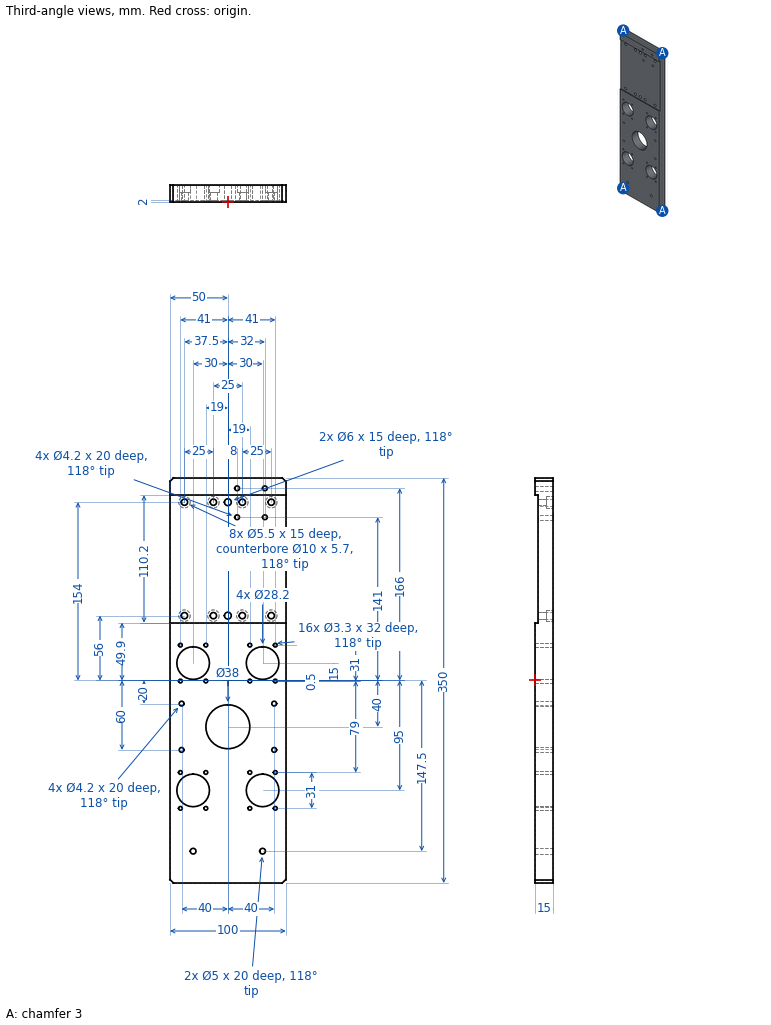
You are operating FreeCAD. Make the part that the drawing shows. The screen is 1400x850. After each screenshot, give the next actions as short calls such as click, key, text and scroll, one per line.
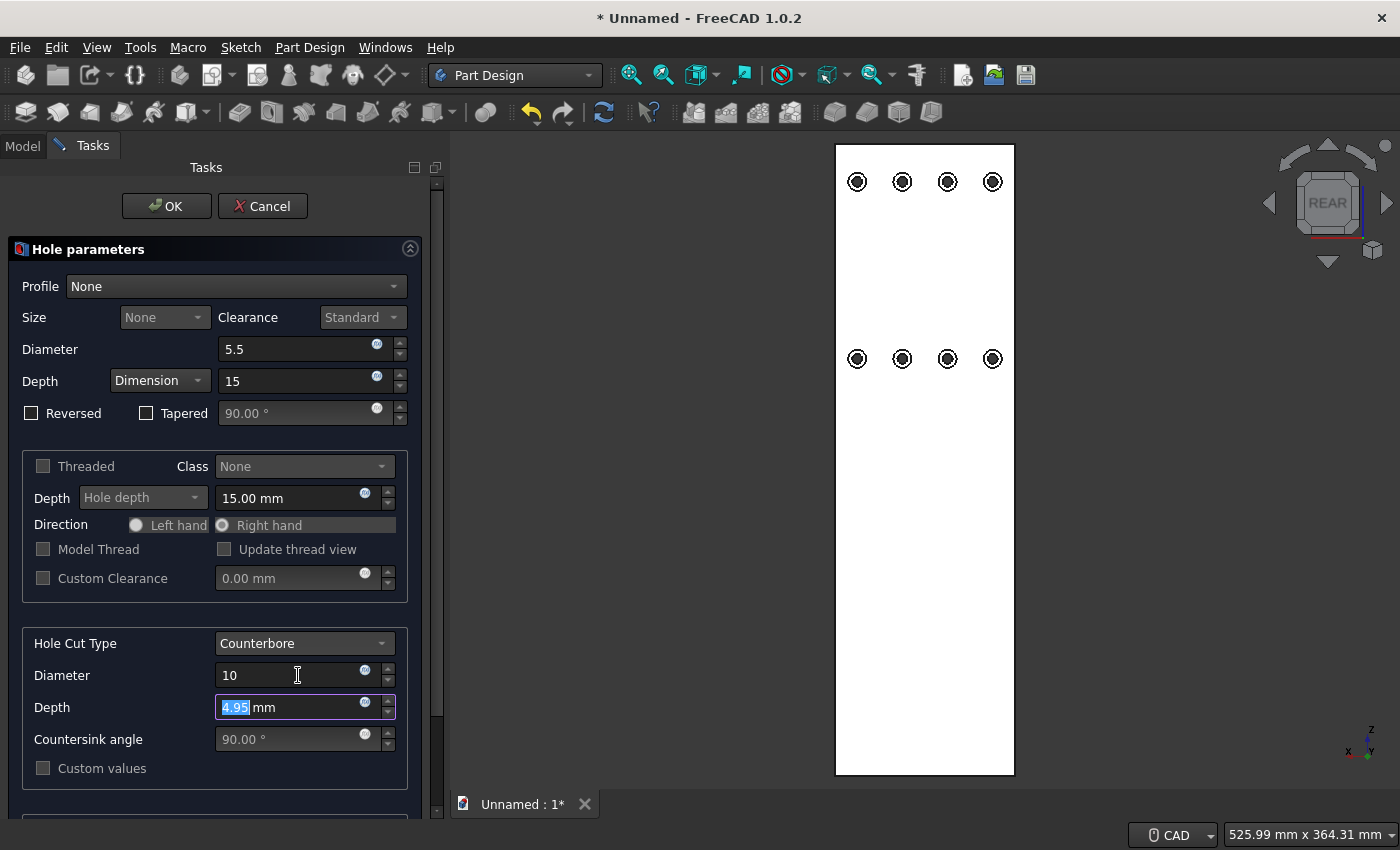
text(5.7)
key(Tab)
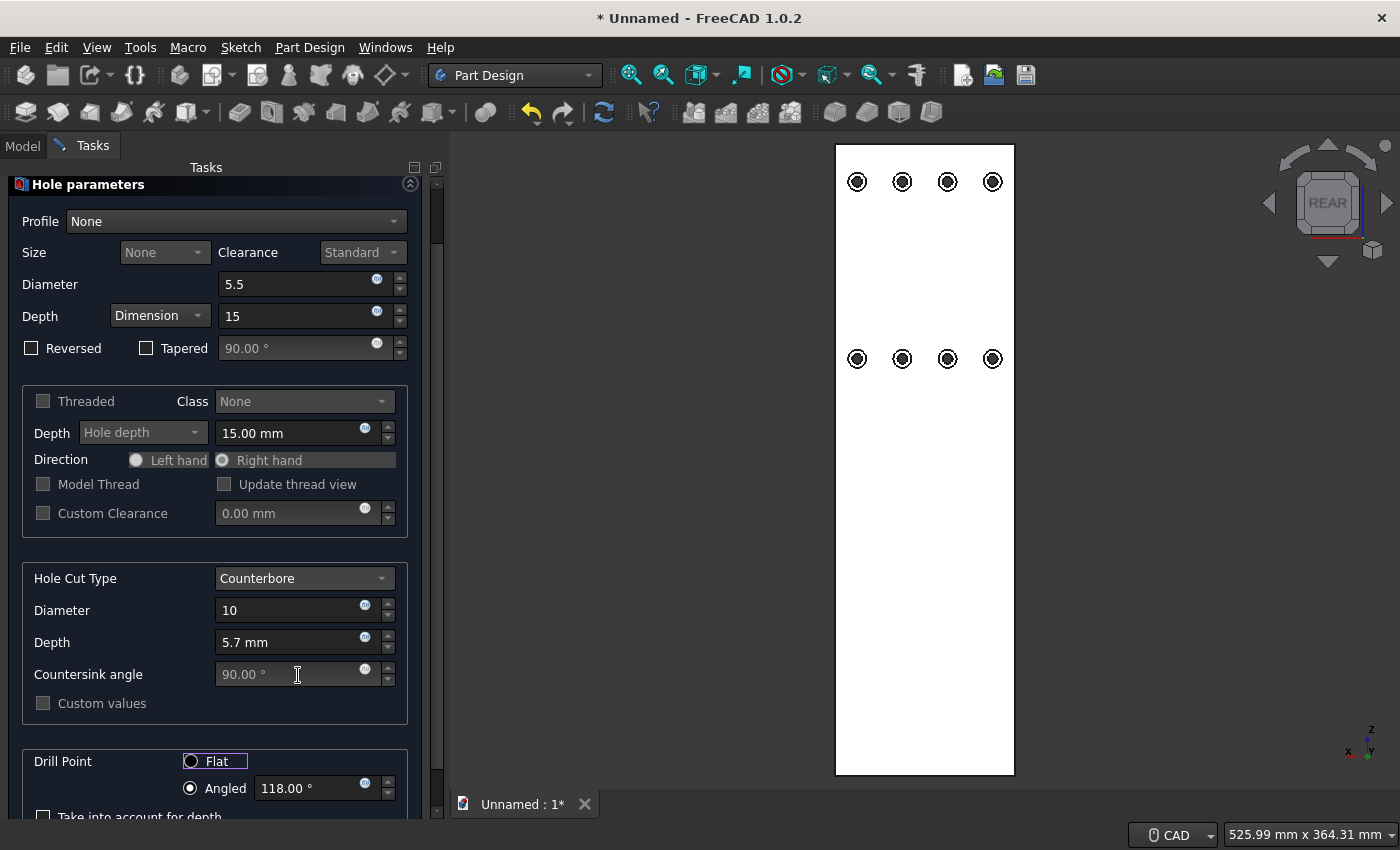
scroll(437, 498, up, 2)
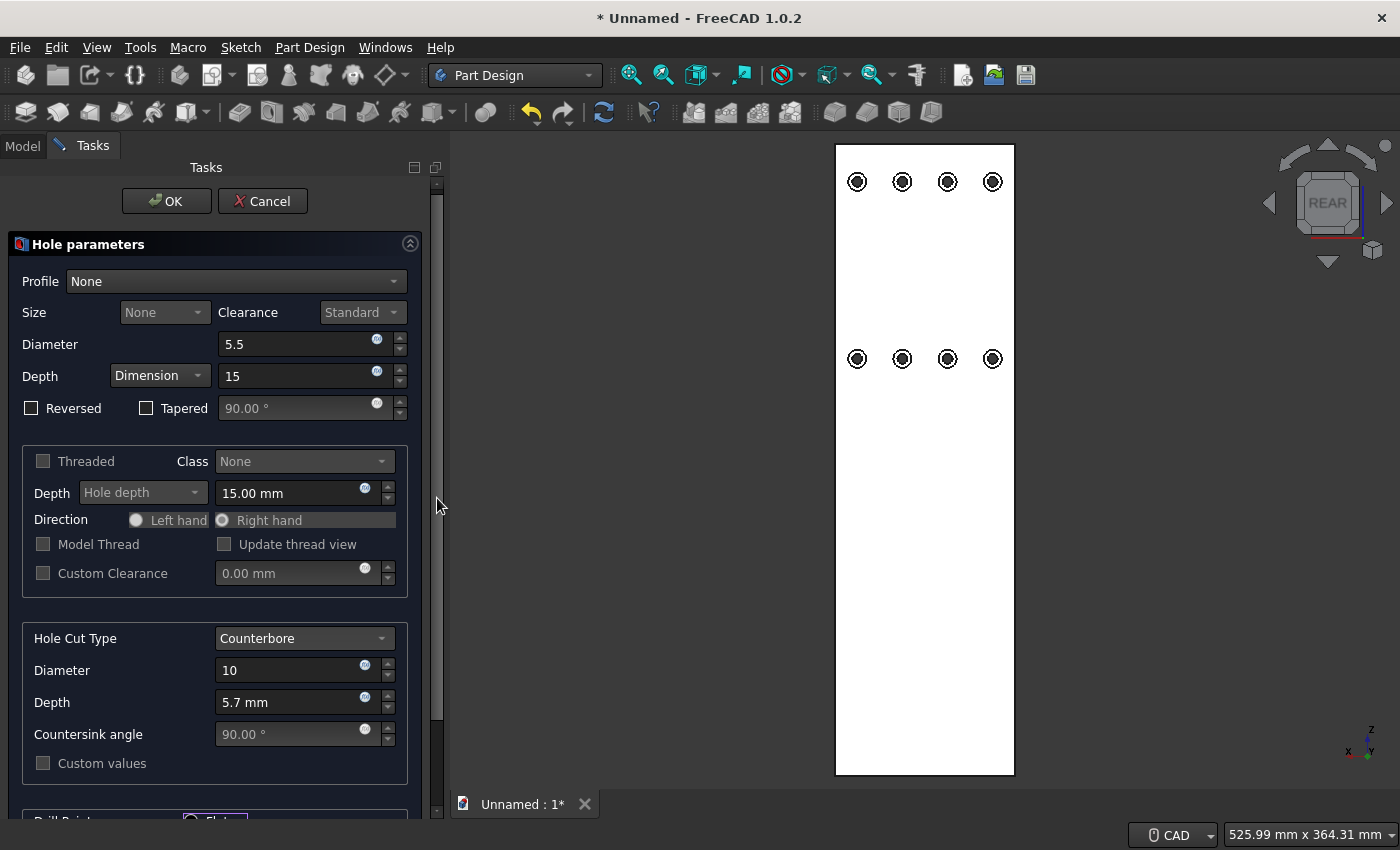
click(167, 206)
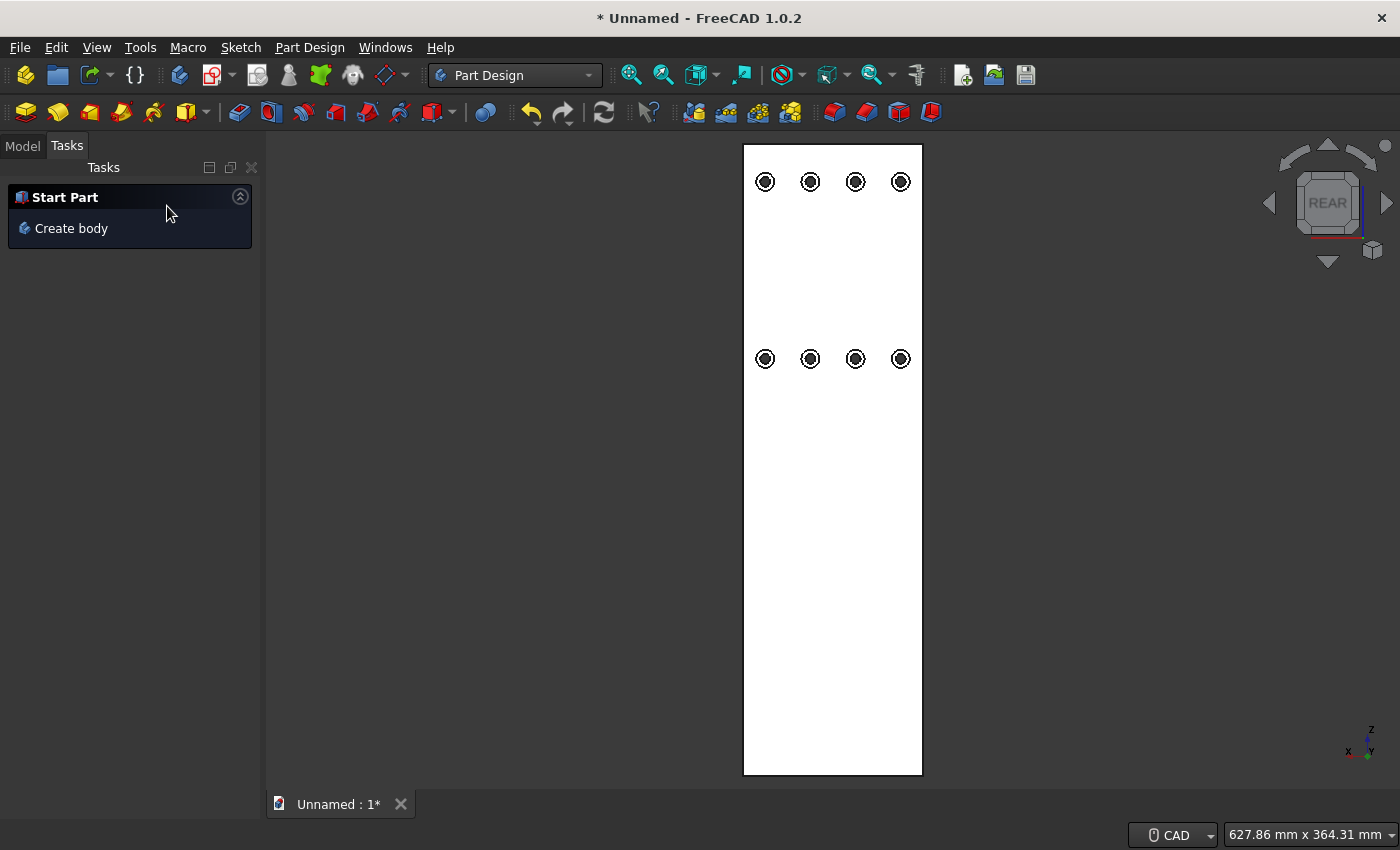
click(833, 459)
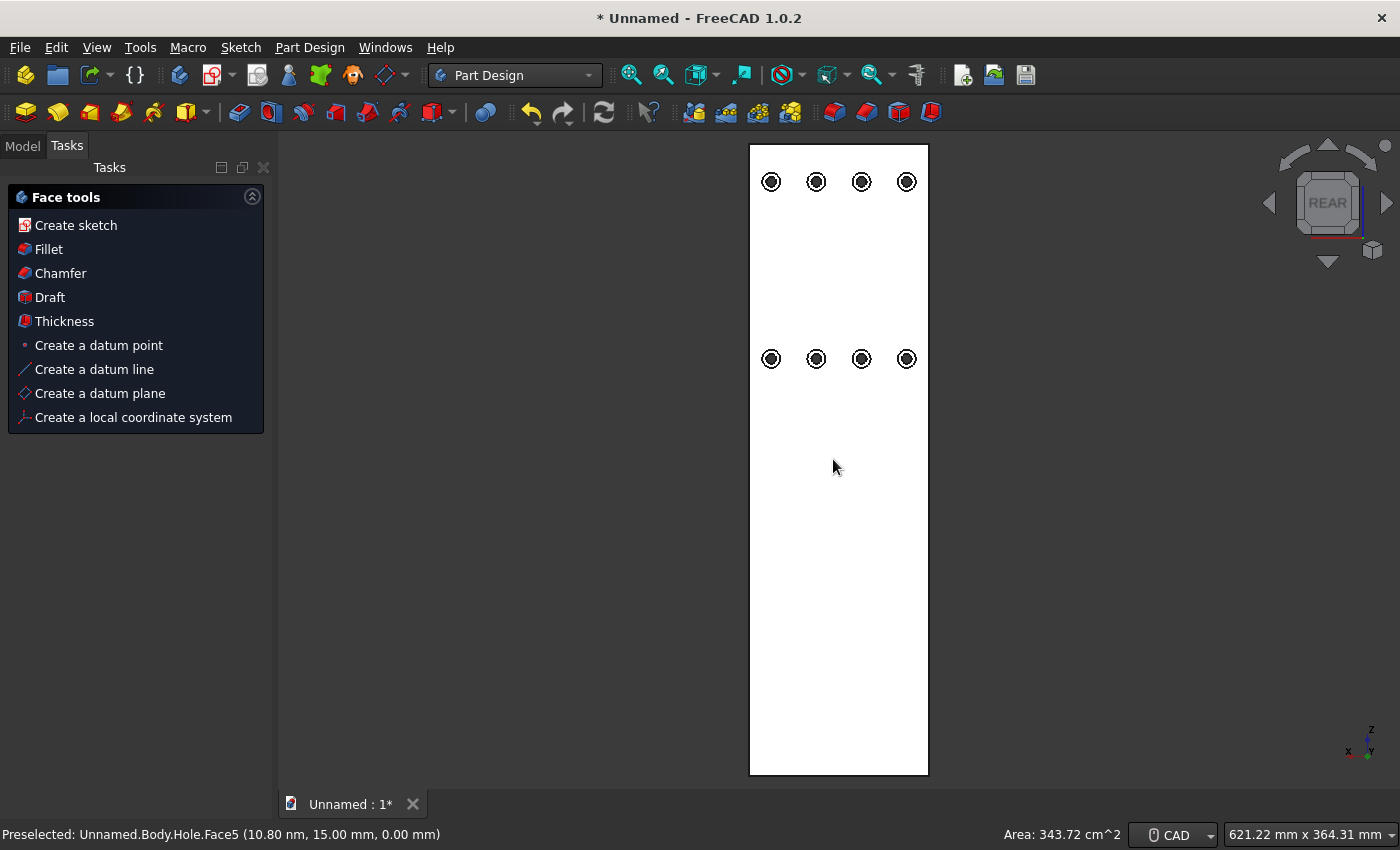
click(212, 76)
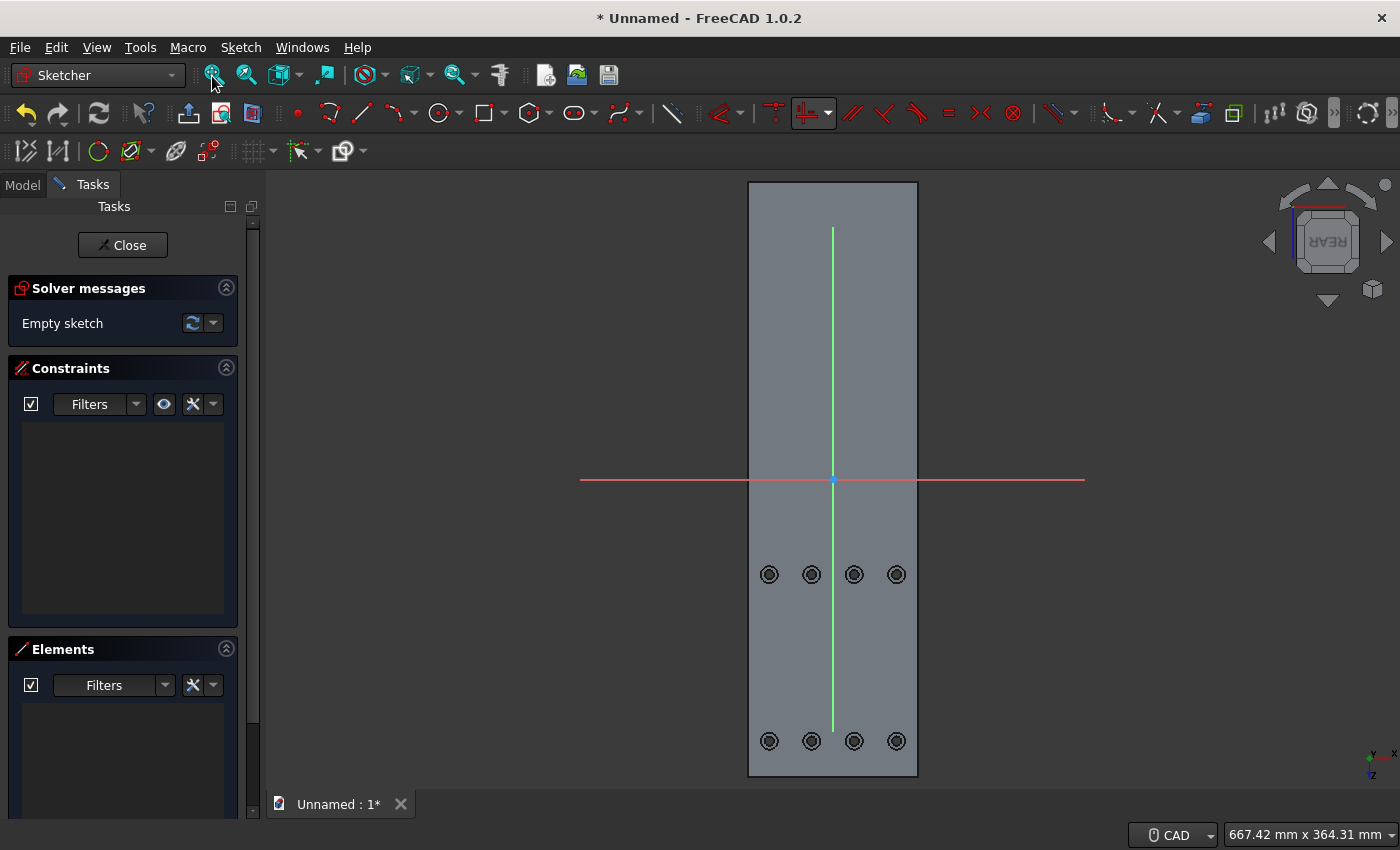
scroll(455, 198, down, 1)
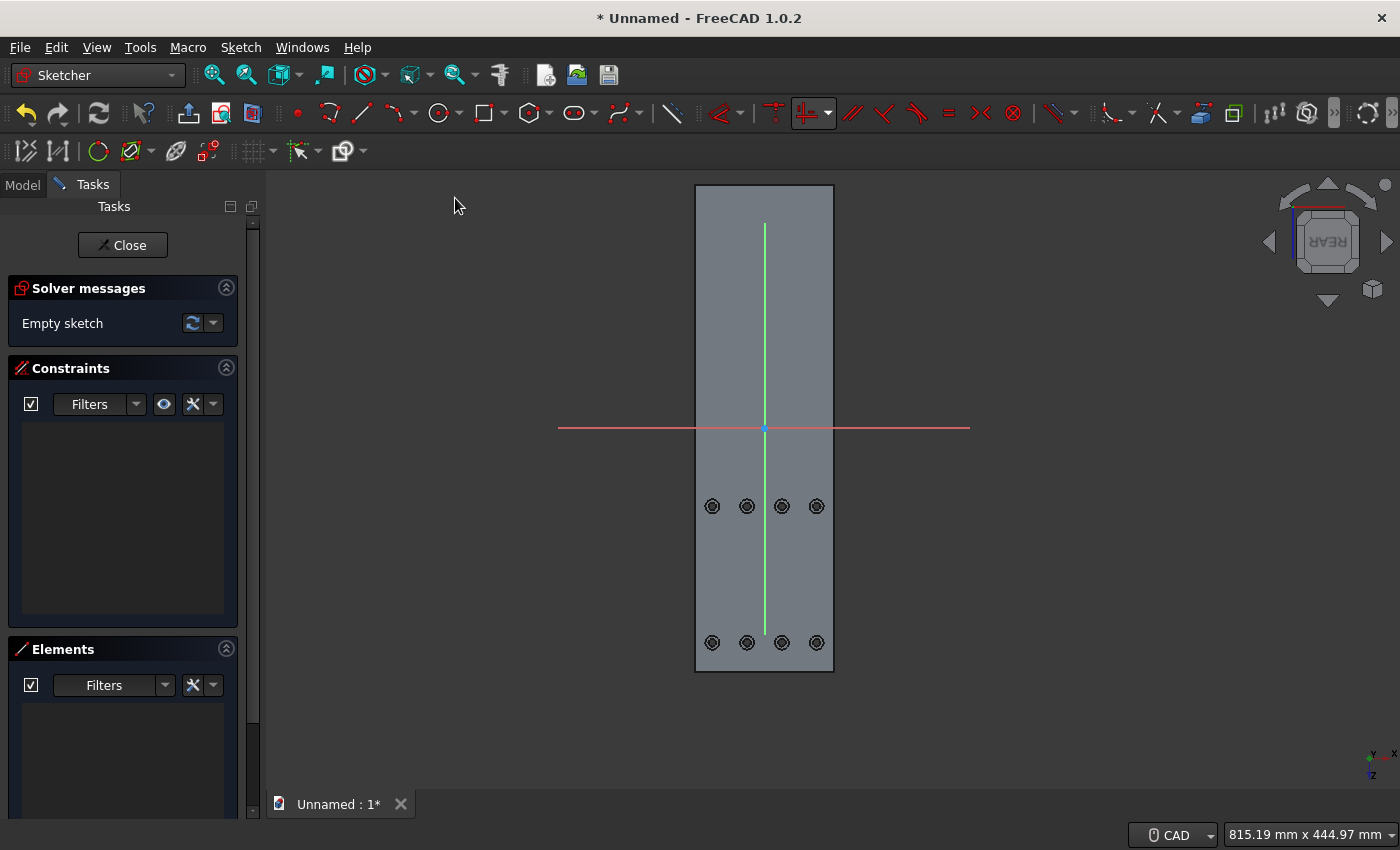
scroll(765, 608, up, 3)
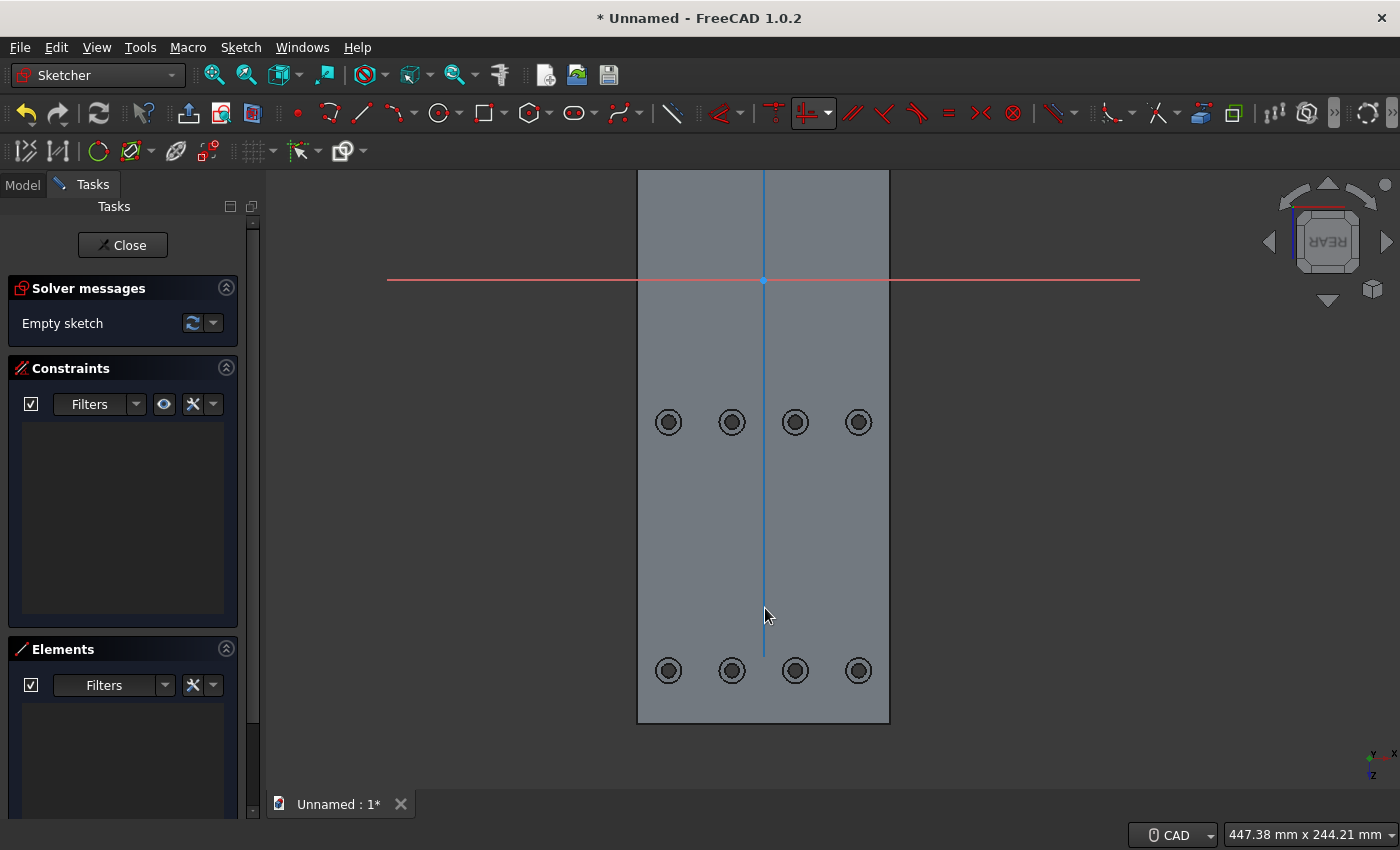
click(440, 114)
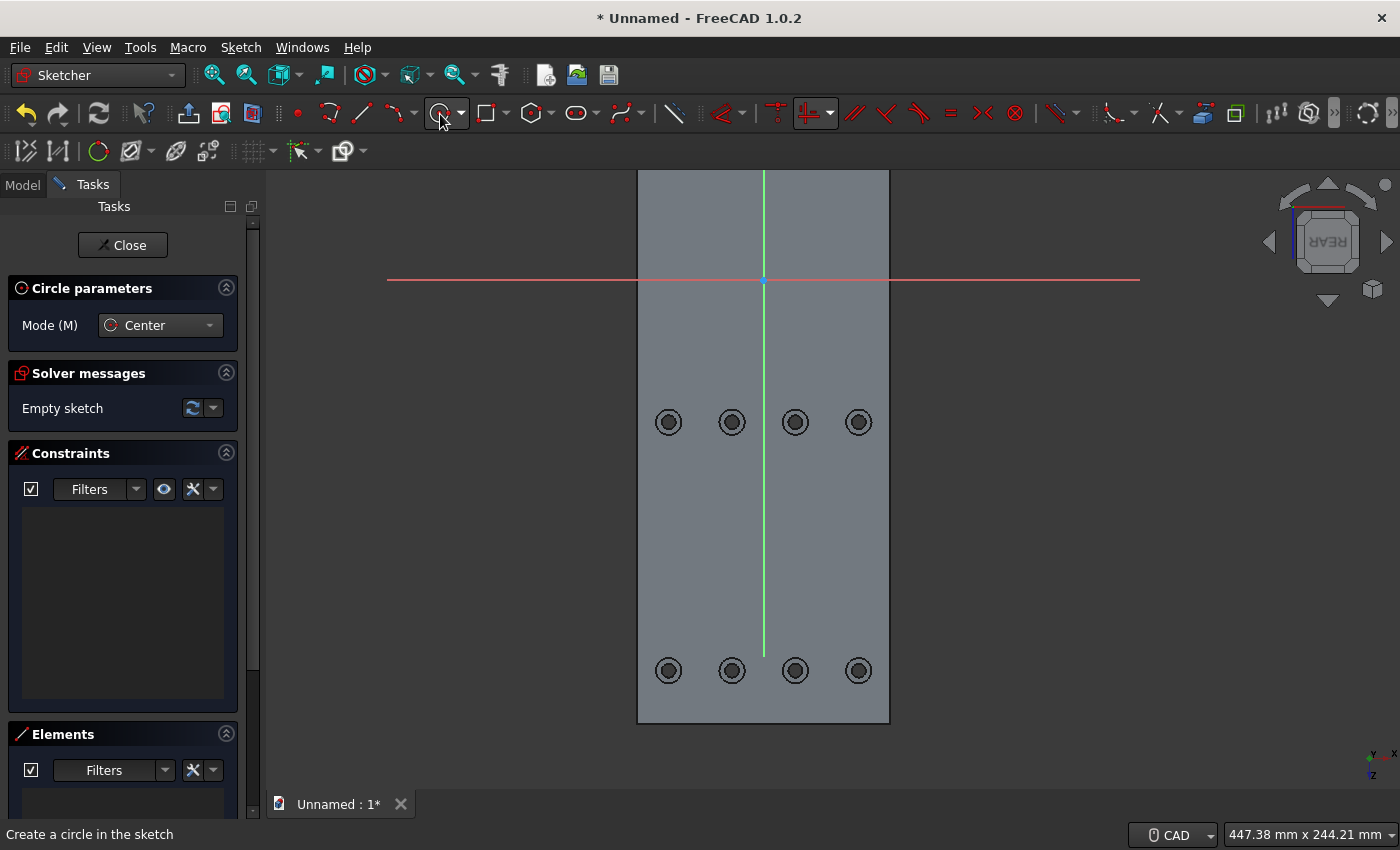
scroll(764, 671, up, 6)